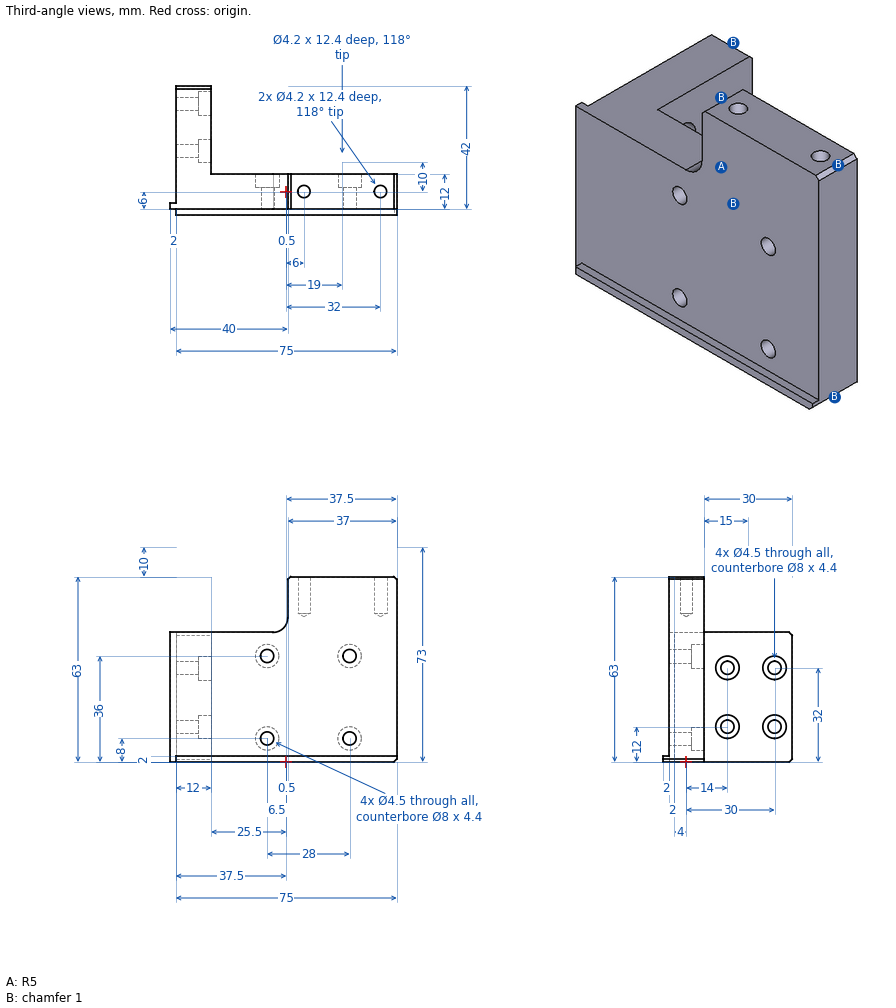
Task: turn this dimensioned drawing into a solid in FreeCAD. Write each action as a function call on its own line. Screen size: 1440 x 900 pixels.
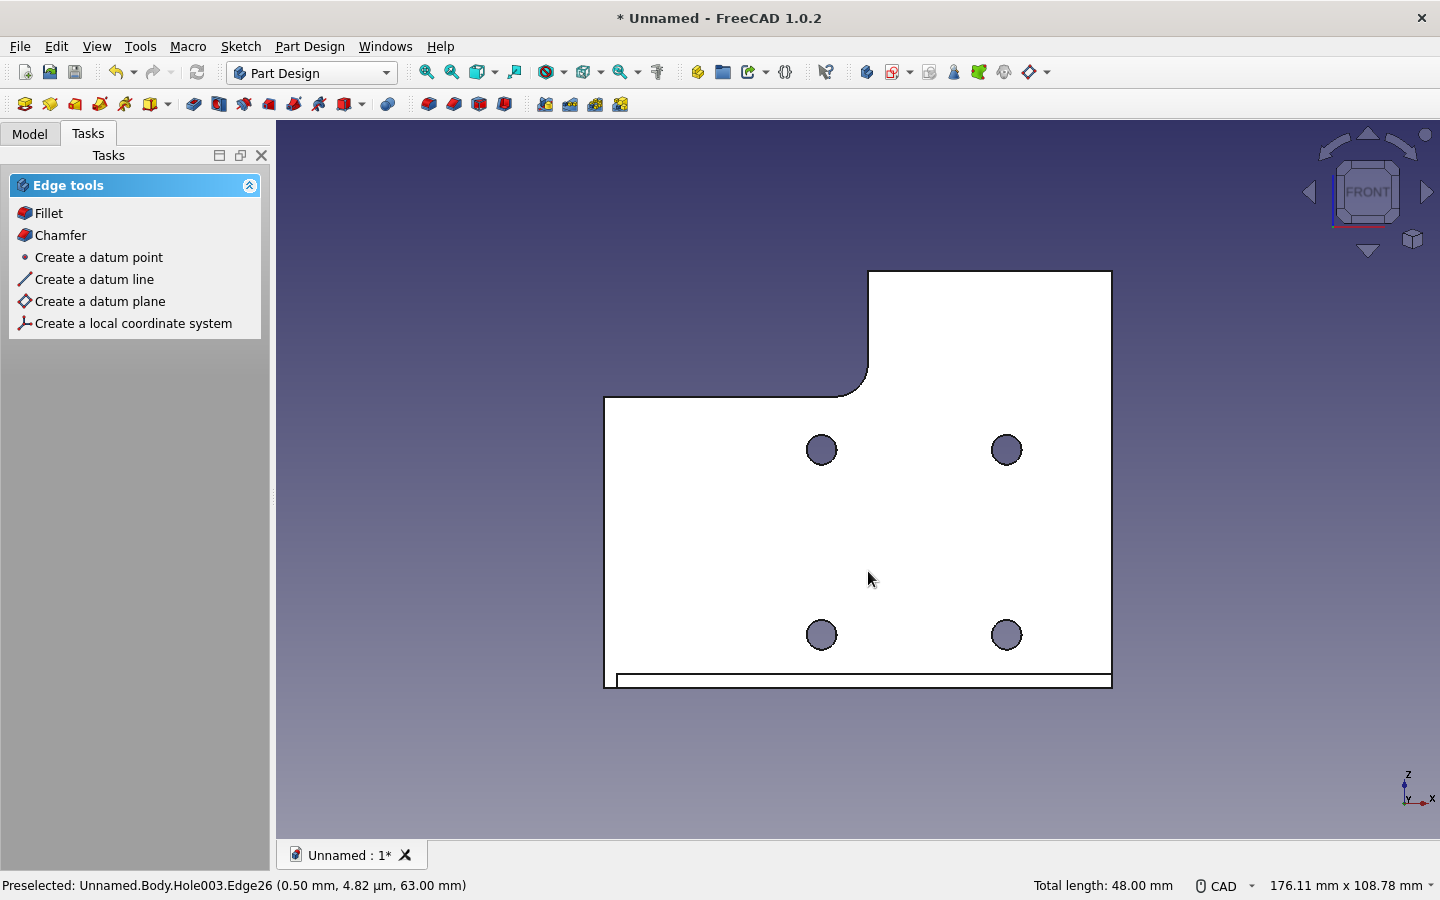
key(3)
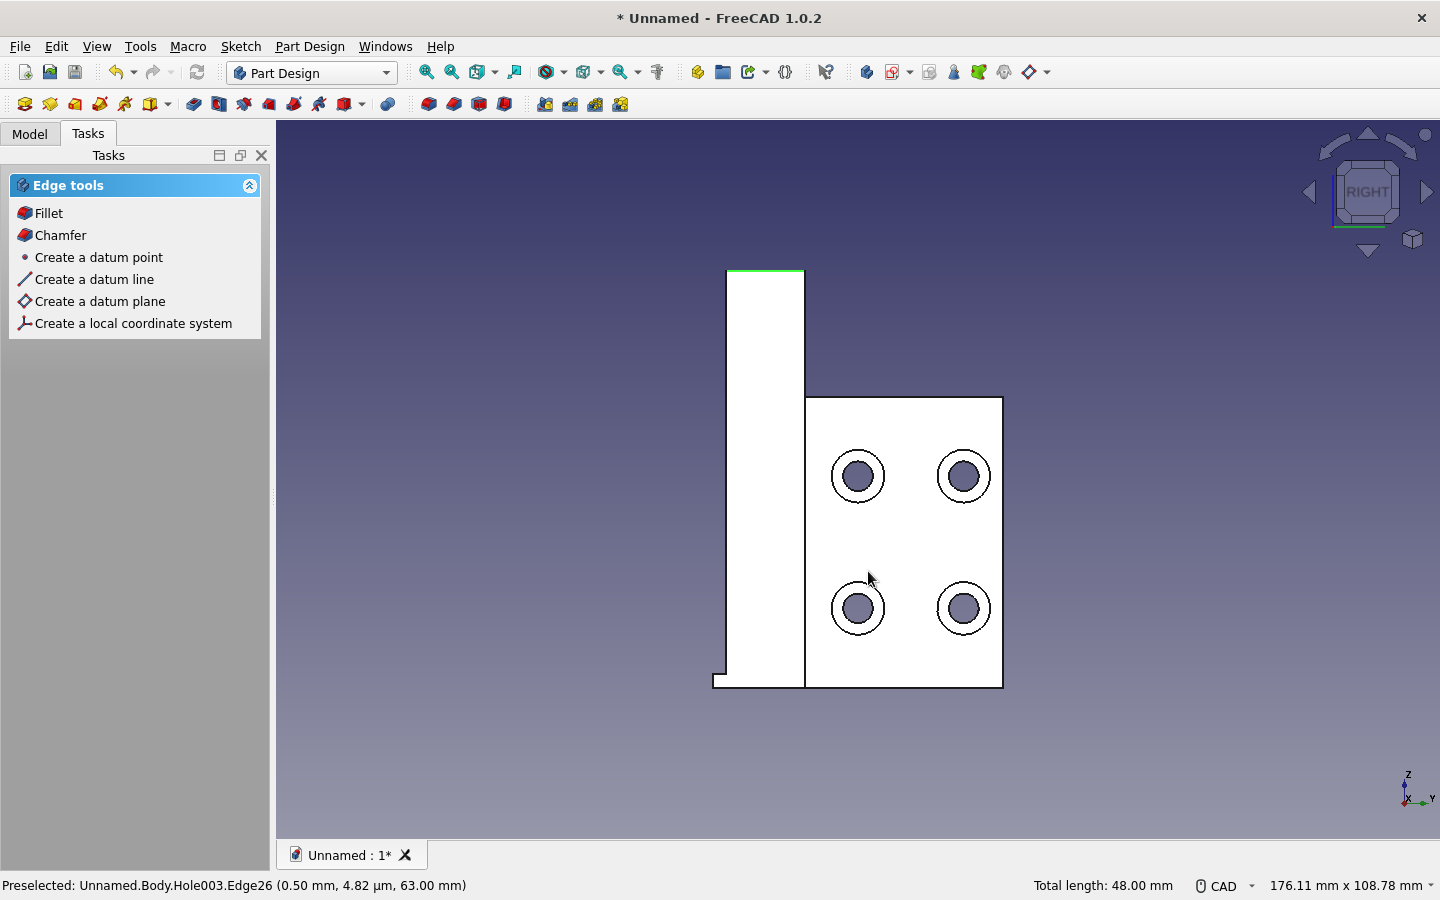
click(759, 687, ctrl)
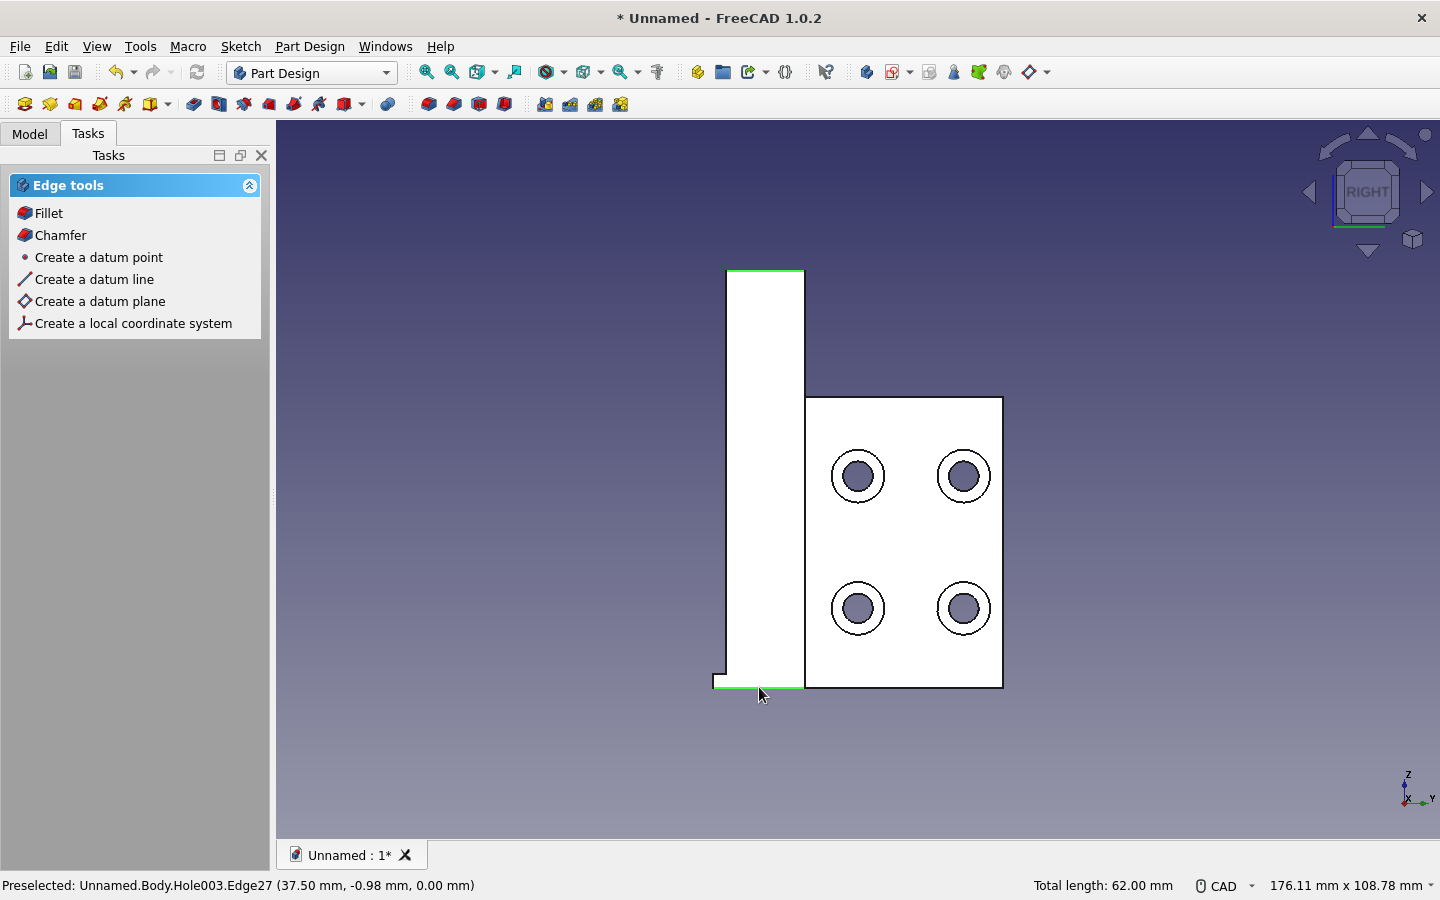
click(454, 104)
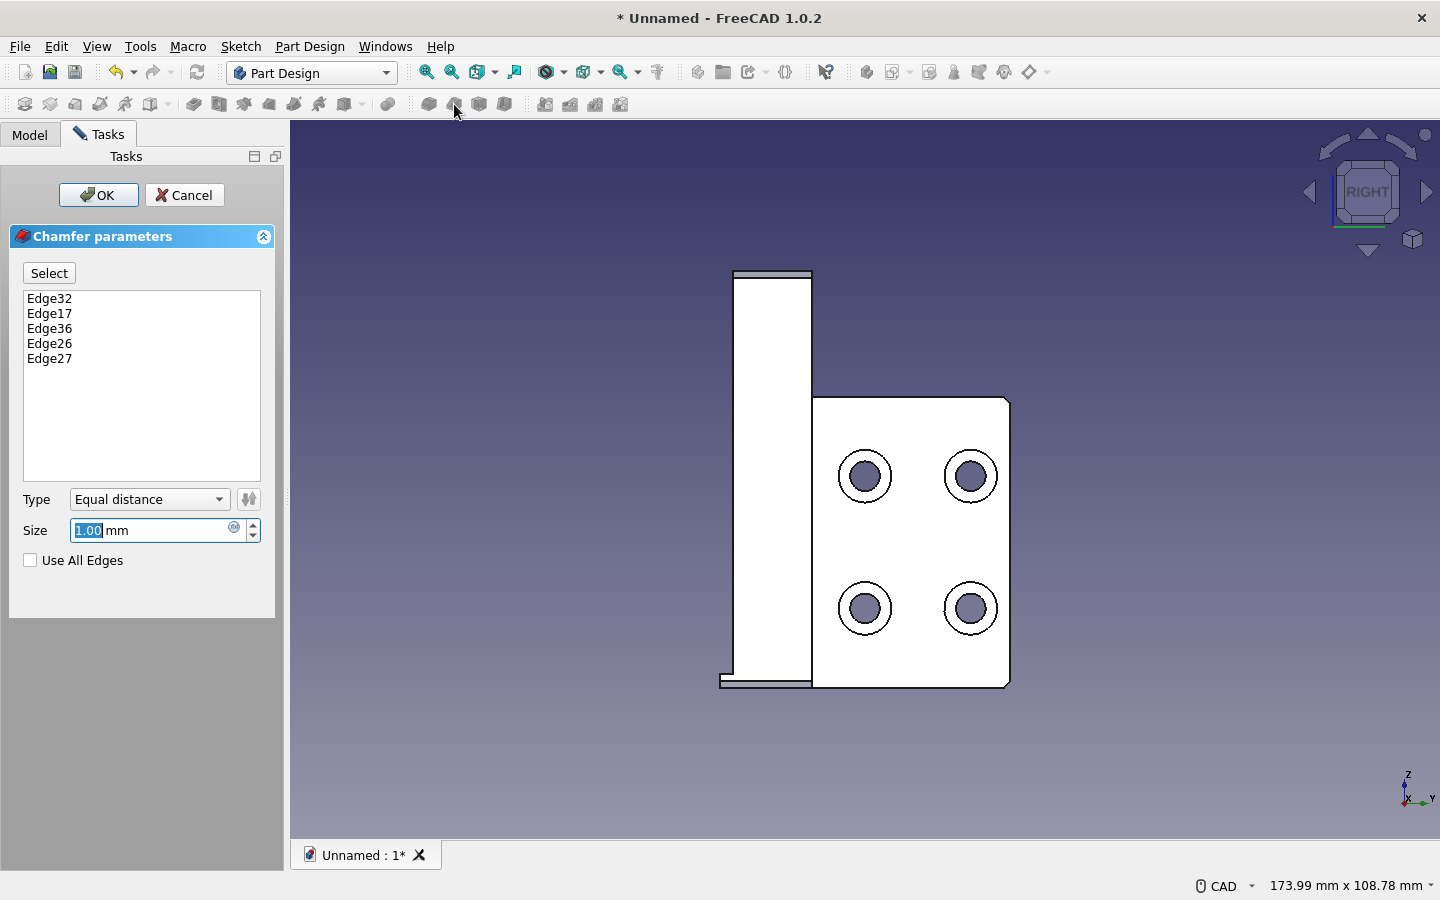
text(1)
key(Tab)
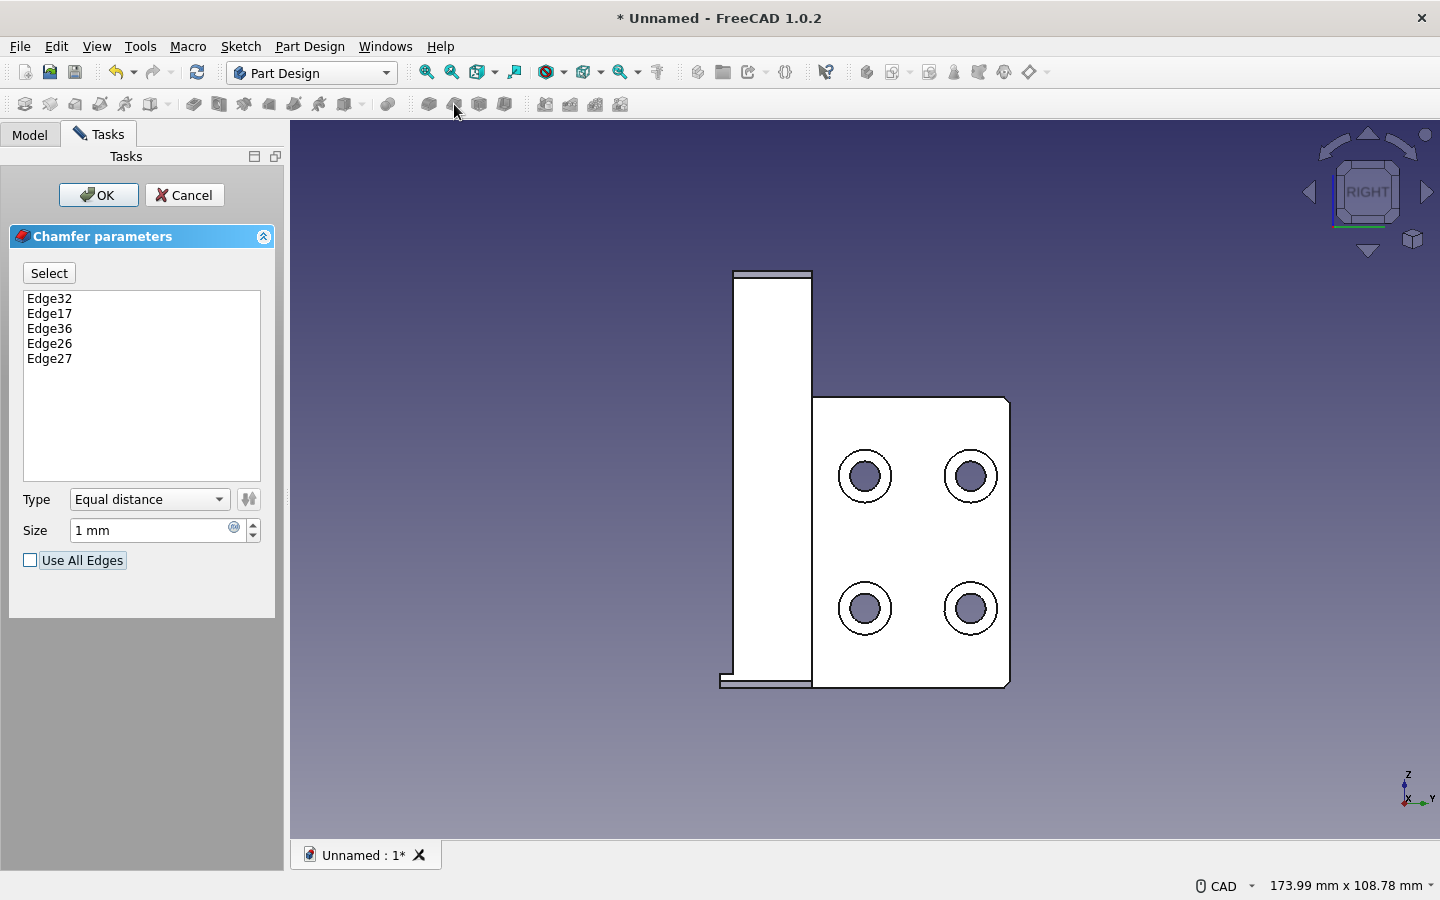
click(99, 195)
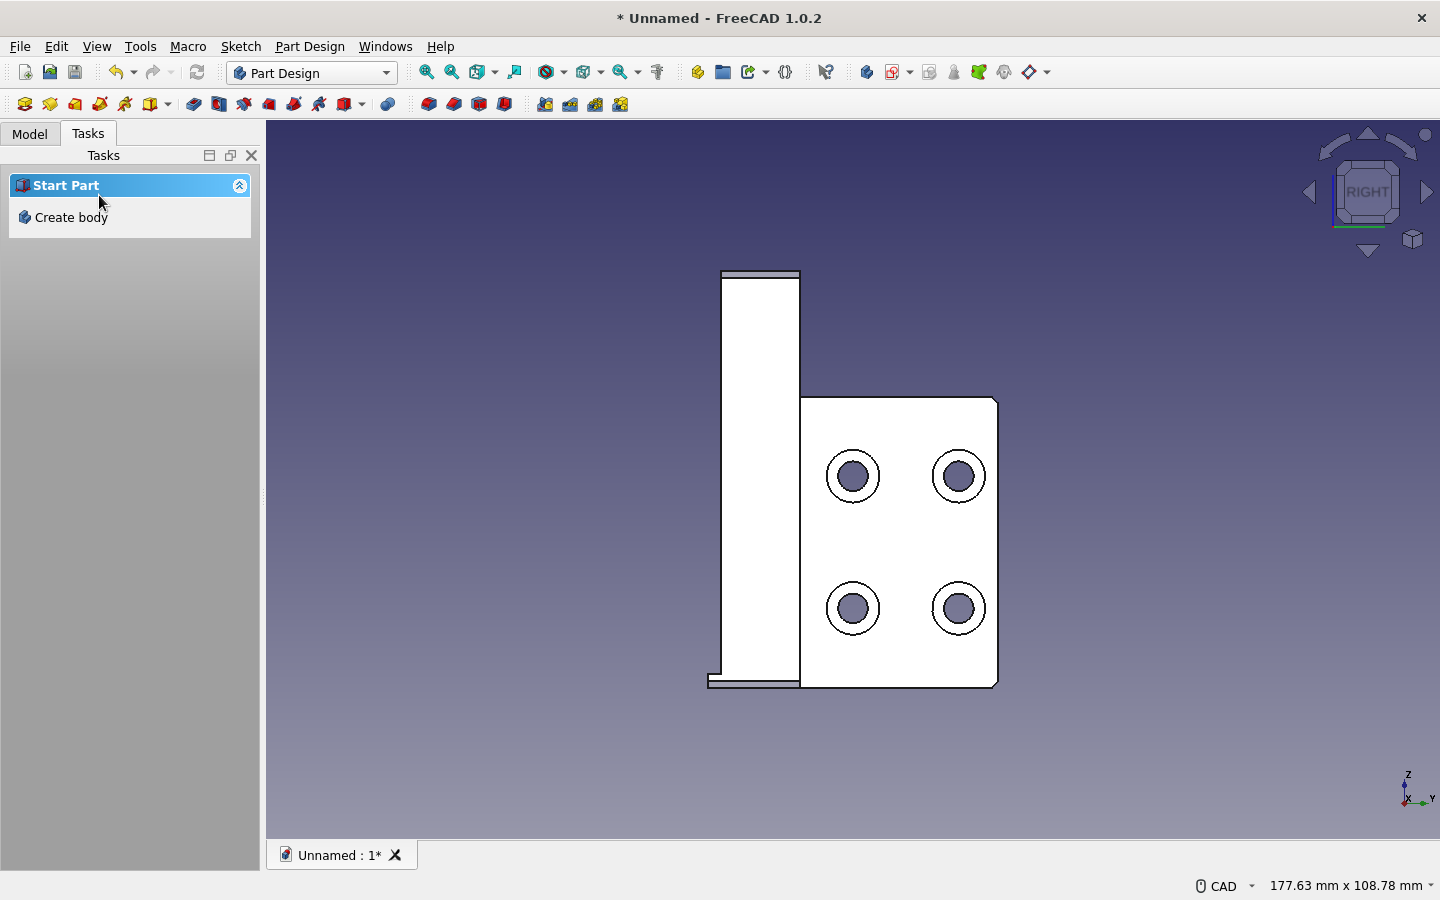
key(0)